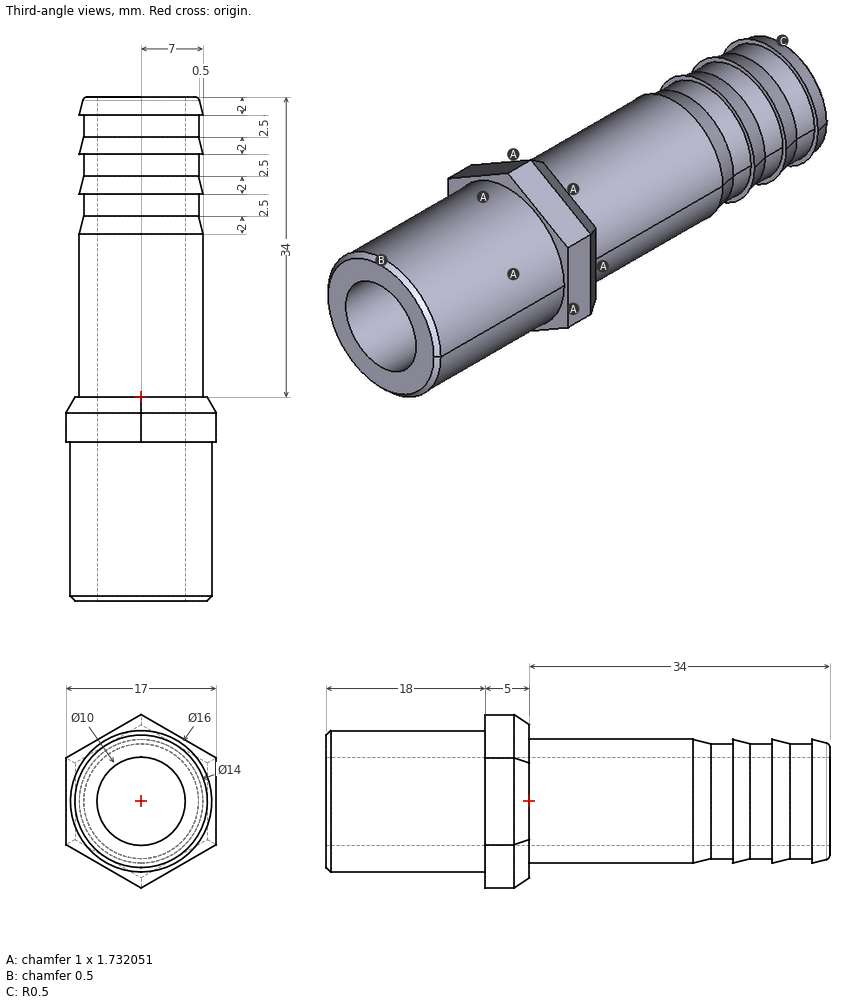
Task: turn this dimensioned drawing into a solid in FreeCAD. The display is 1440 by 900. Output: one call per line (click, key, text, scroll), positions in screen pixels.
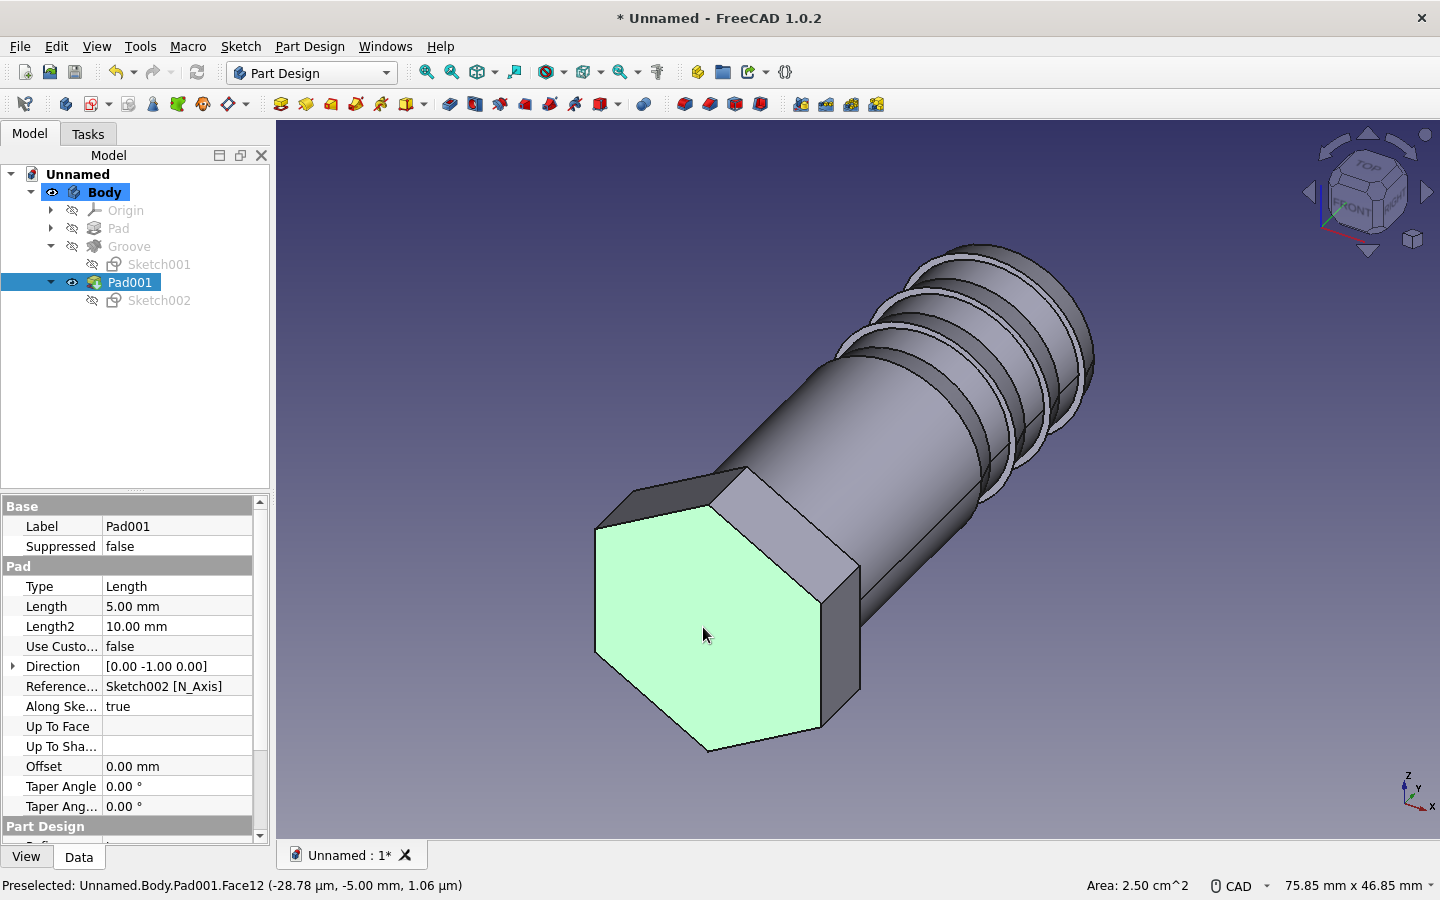
click(90, 104)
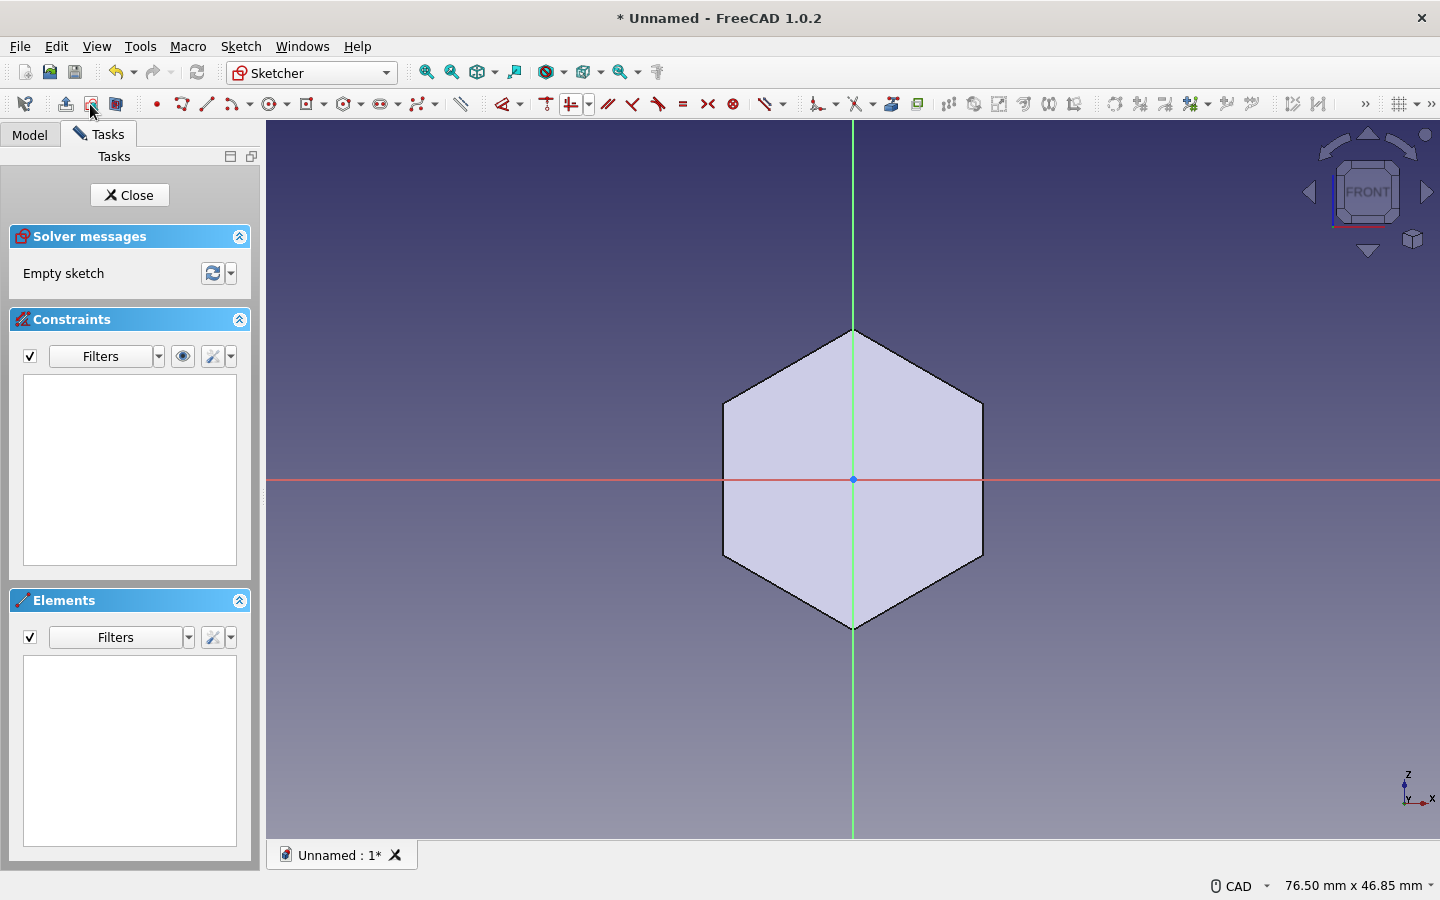
scroll(936, 480, up, 3)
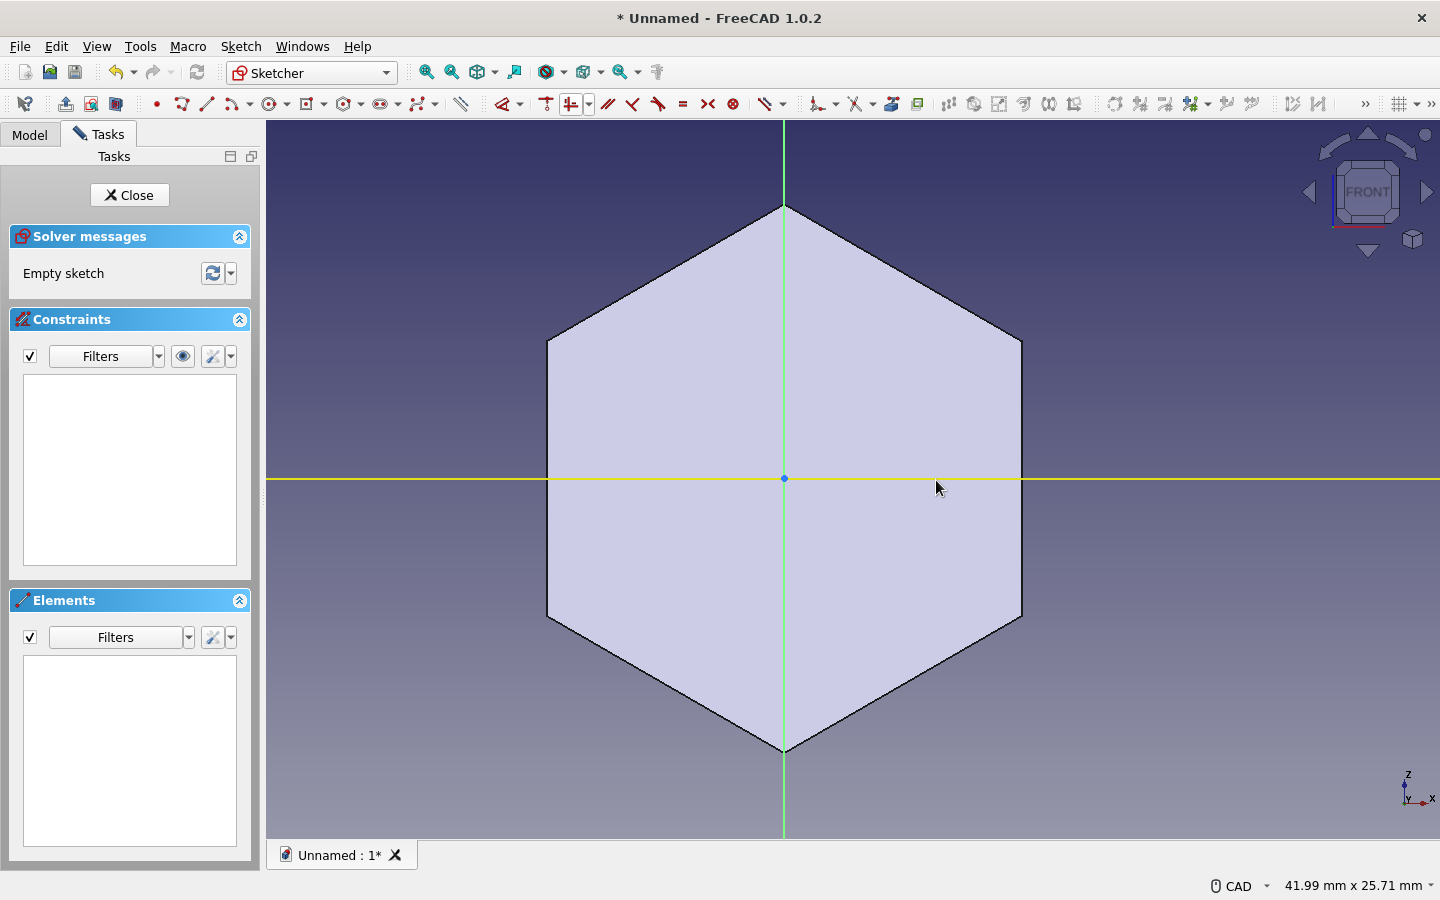
click(268, 104)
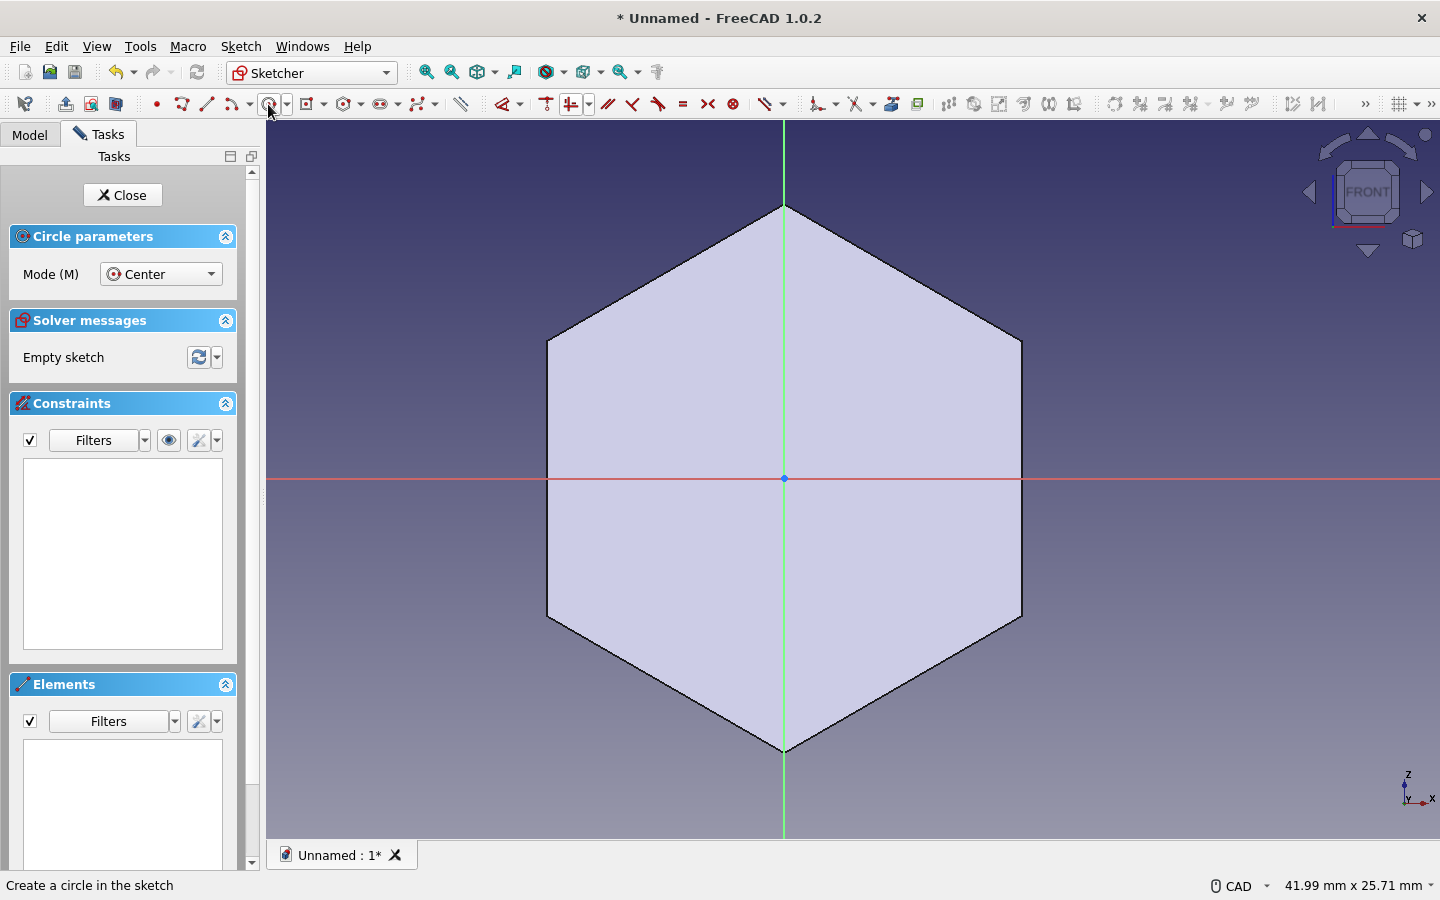
click(784, 479)
click(942, 321)
key(Escape)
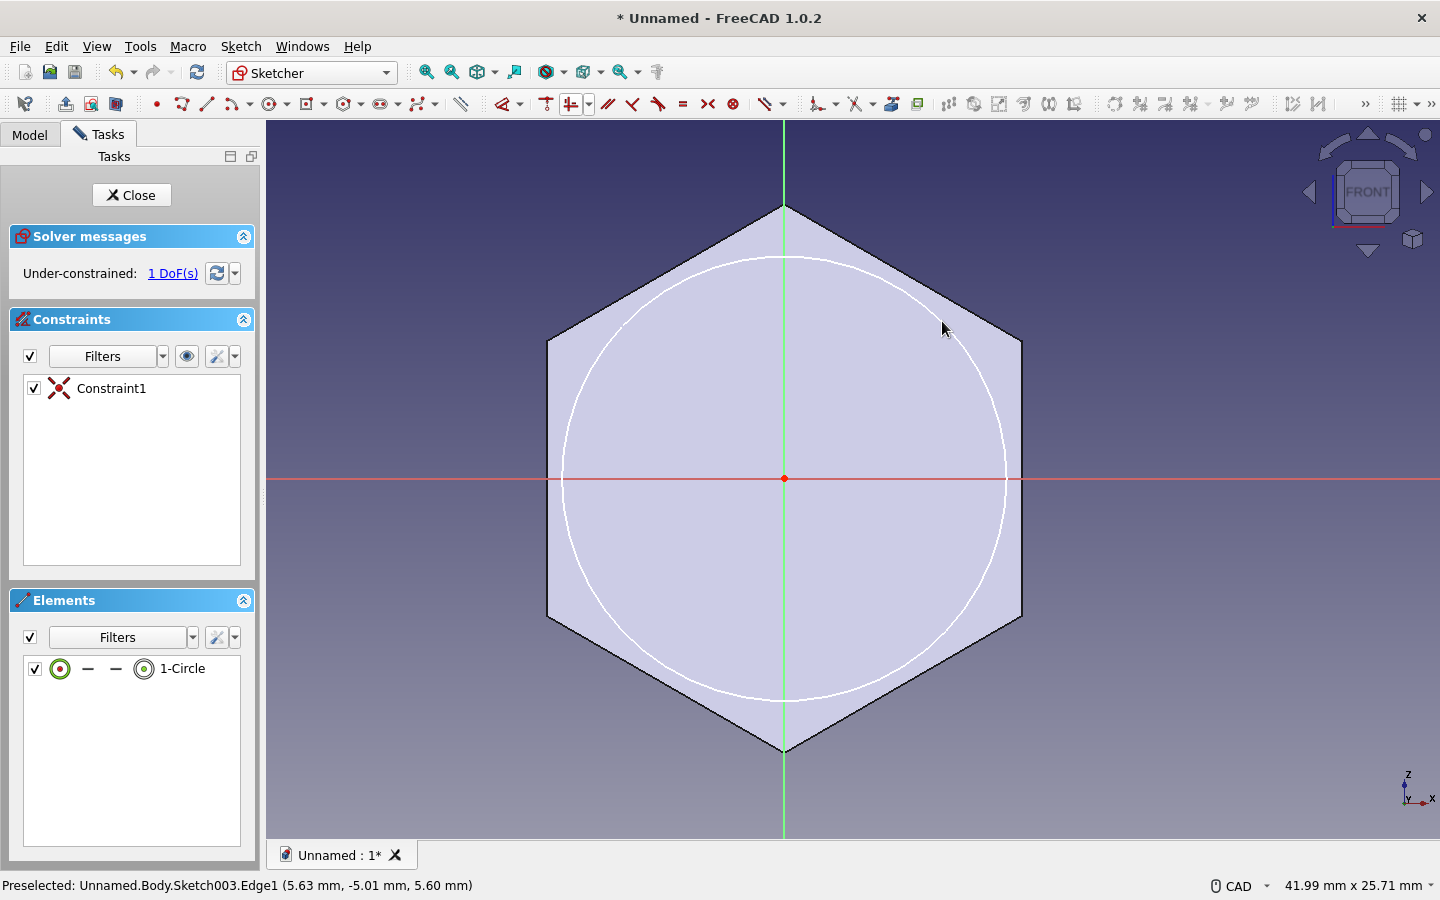
click(502, 104)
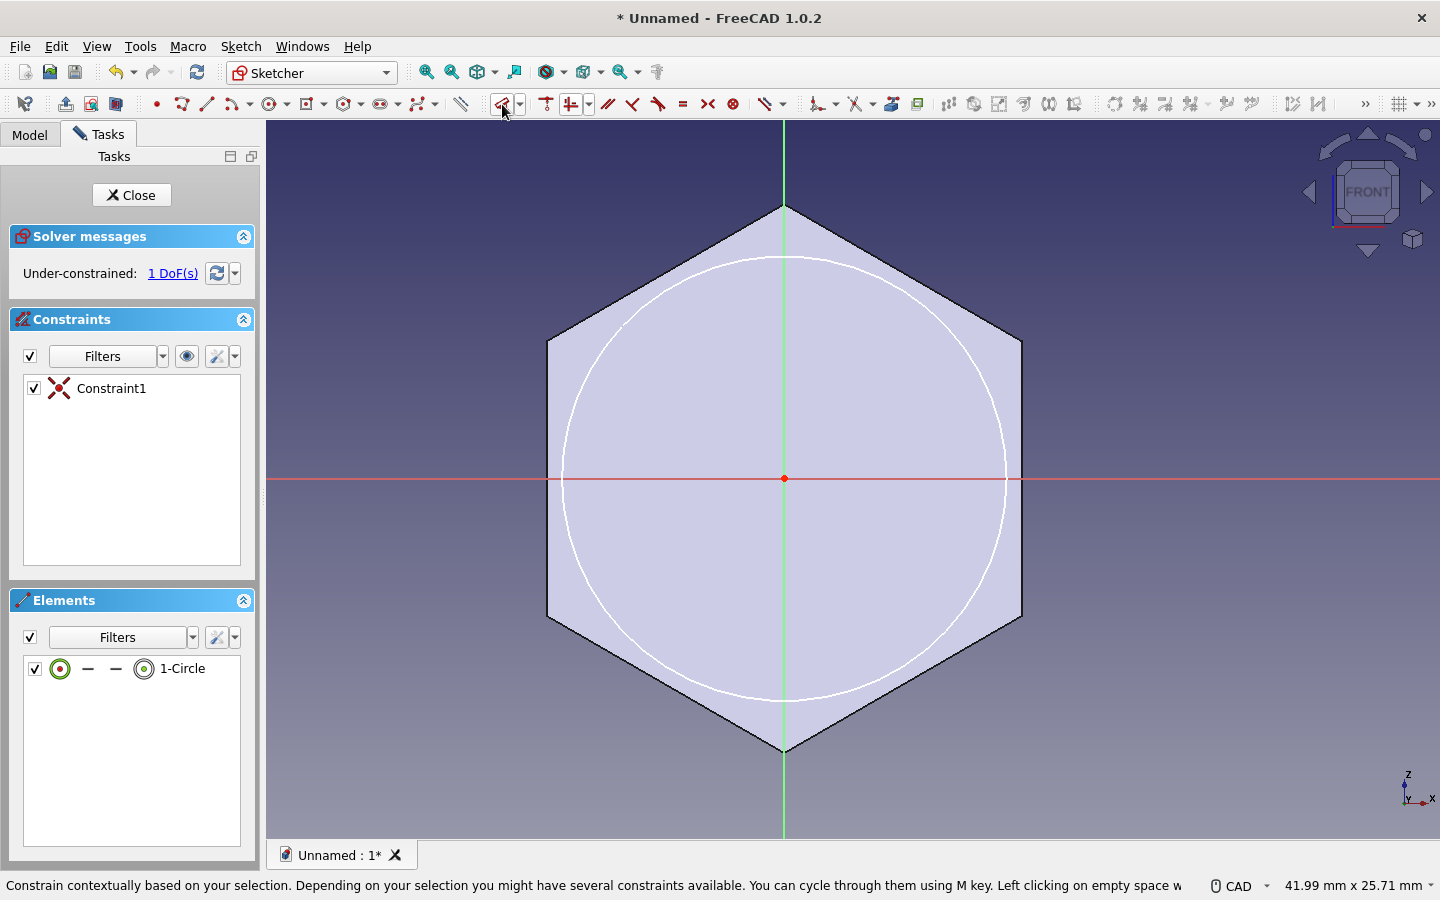
click(941, 321)
click(964, 298)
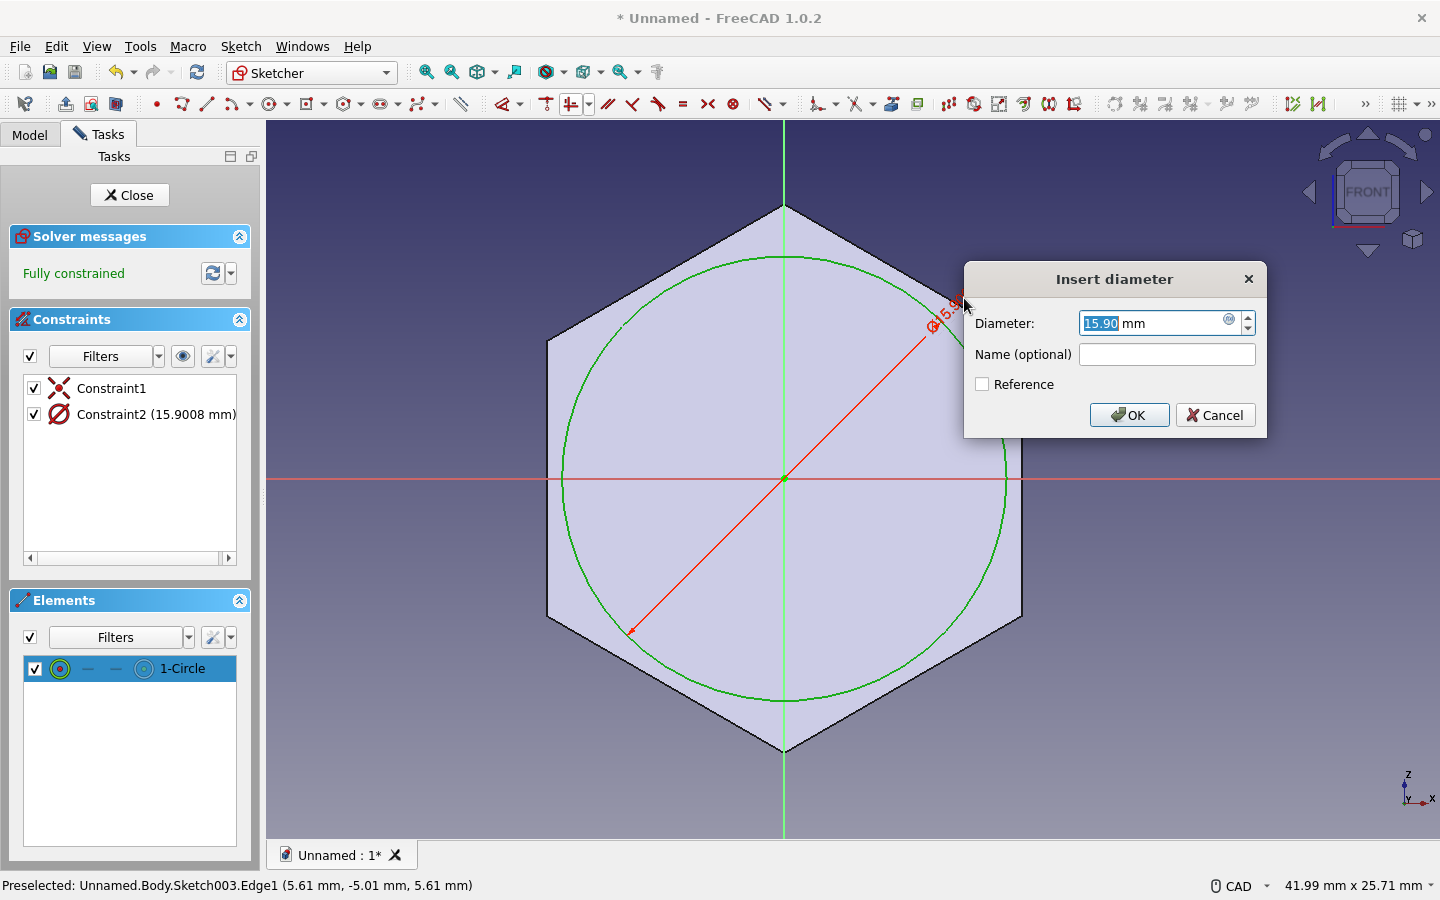
text(16)
key(Return)
key(Escape)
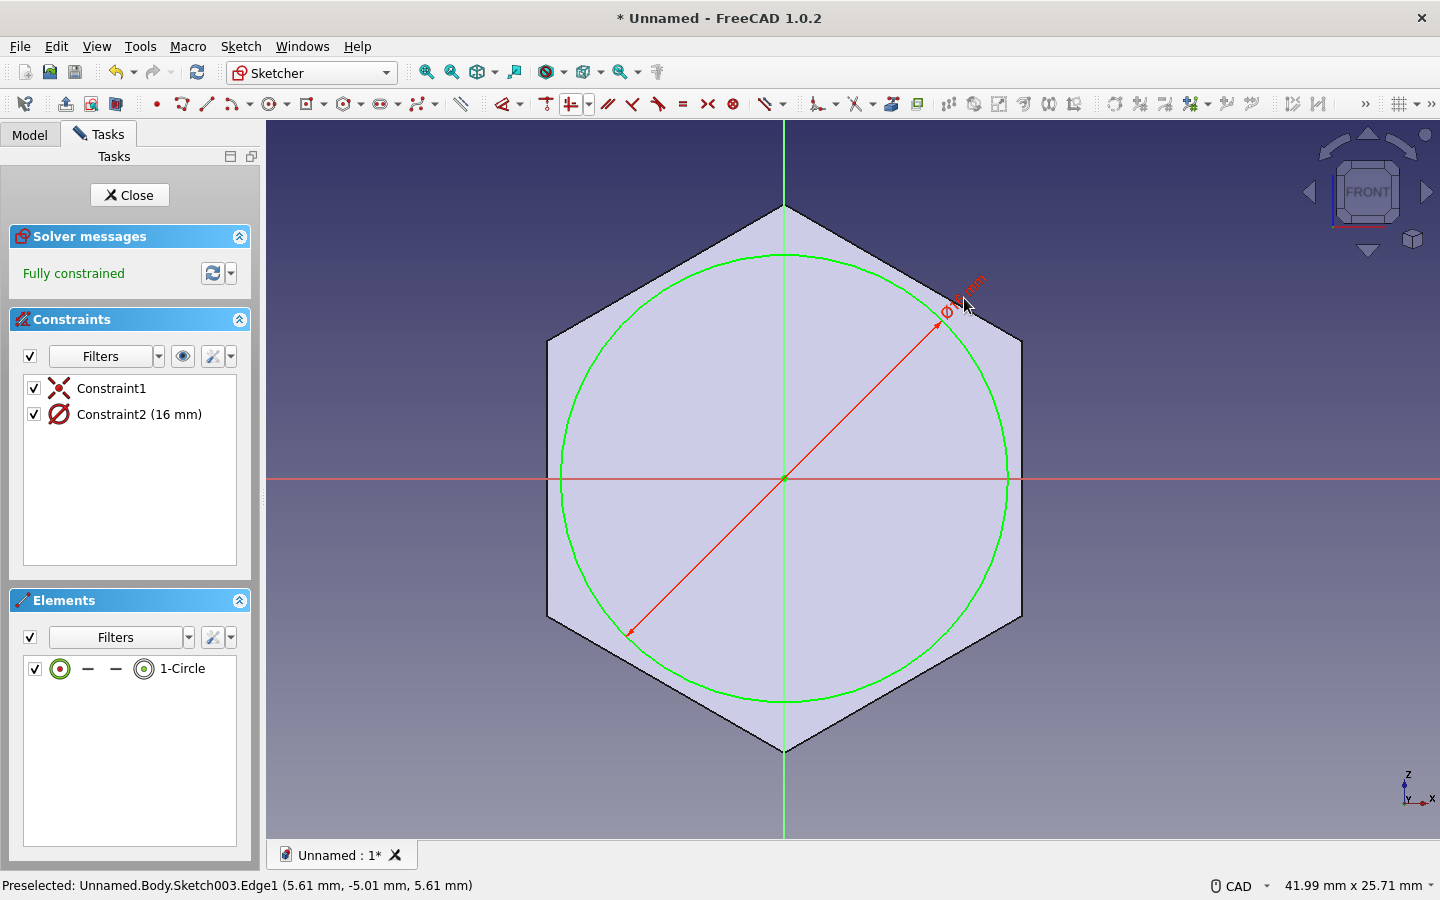
click(130, 195)